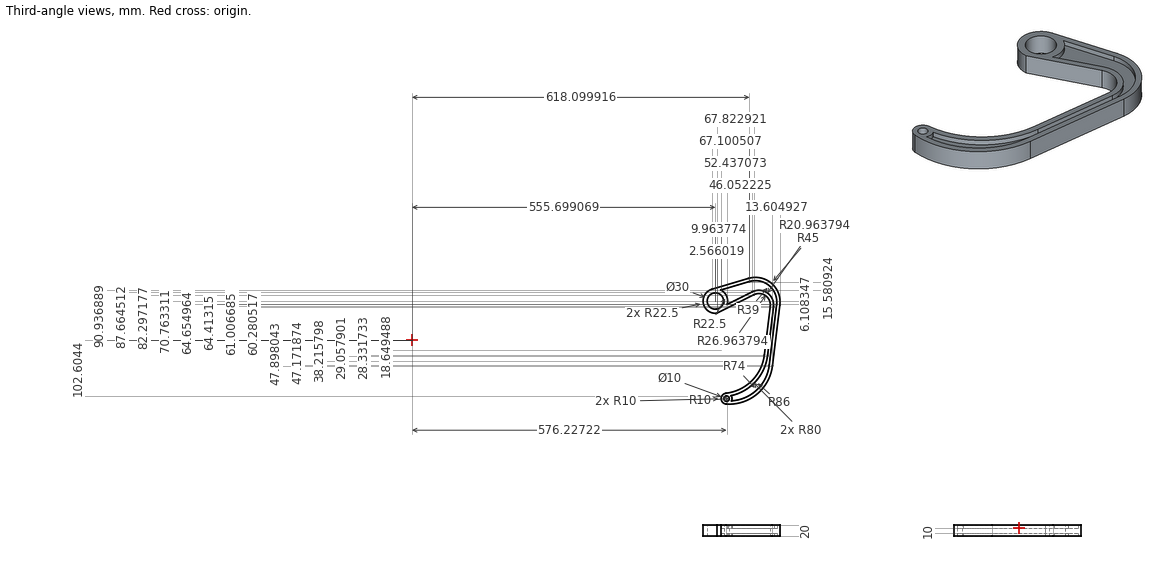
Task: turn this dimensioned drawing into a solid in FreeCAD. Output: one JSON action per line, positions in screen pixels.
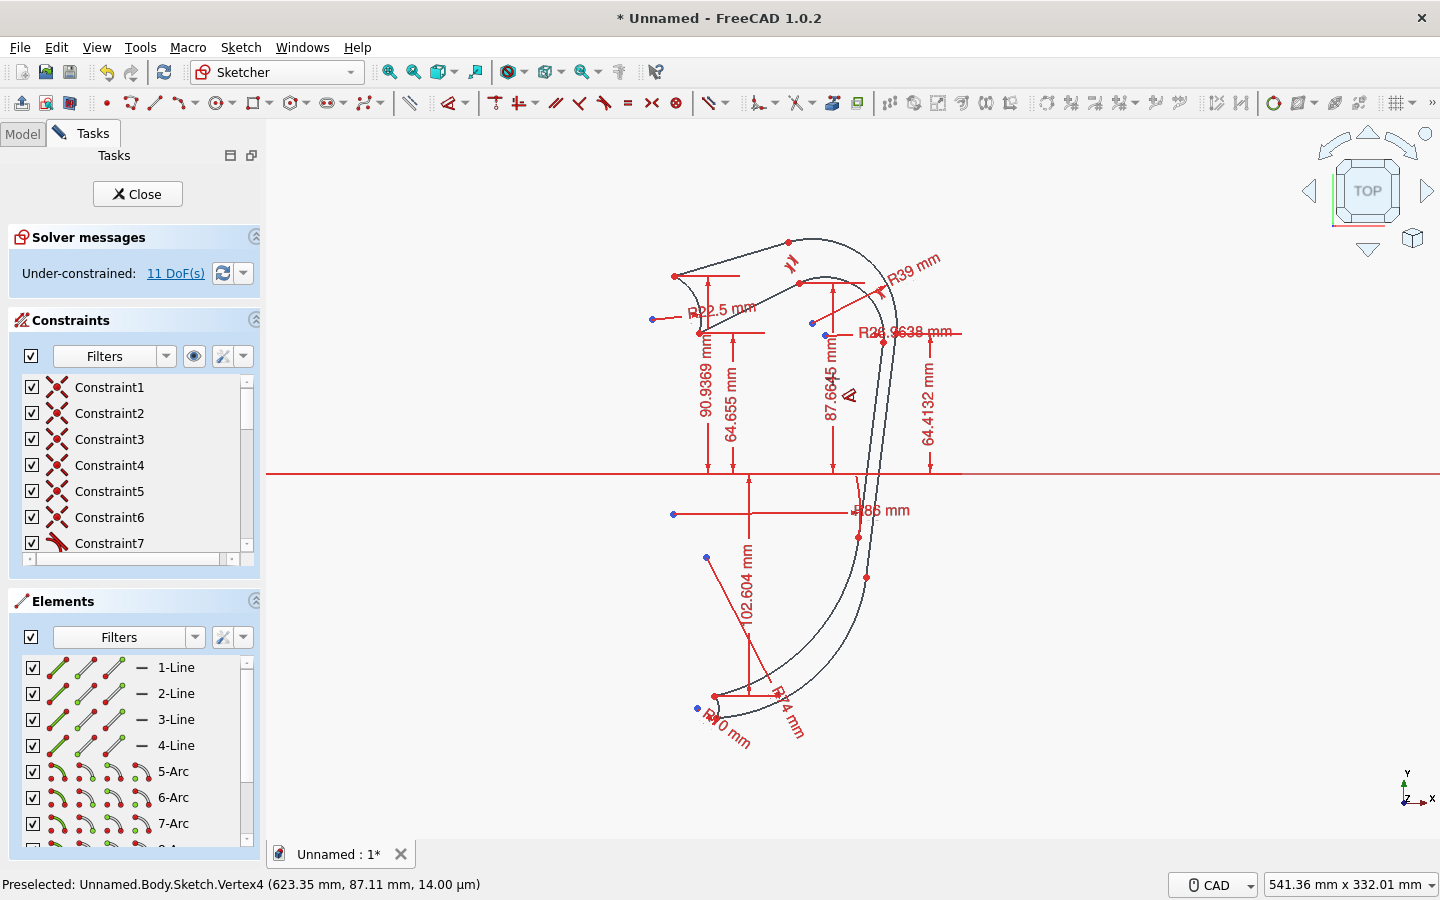
{"action": "left_click", "coordinate": [883, 343]}
{"action": "left_click", "coordinate": [917, 378]}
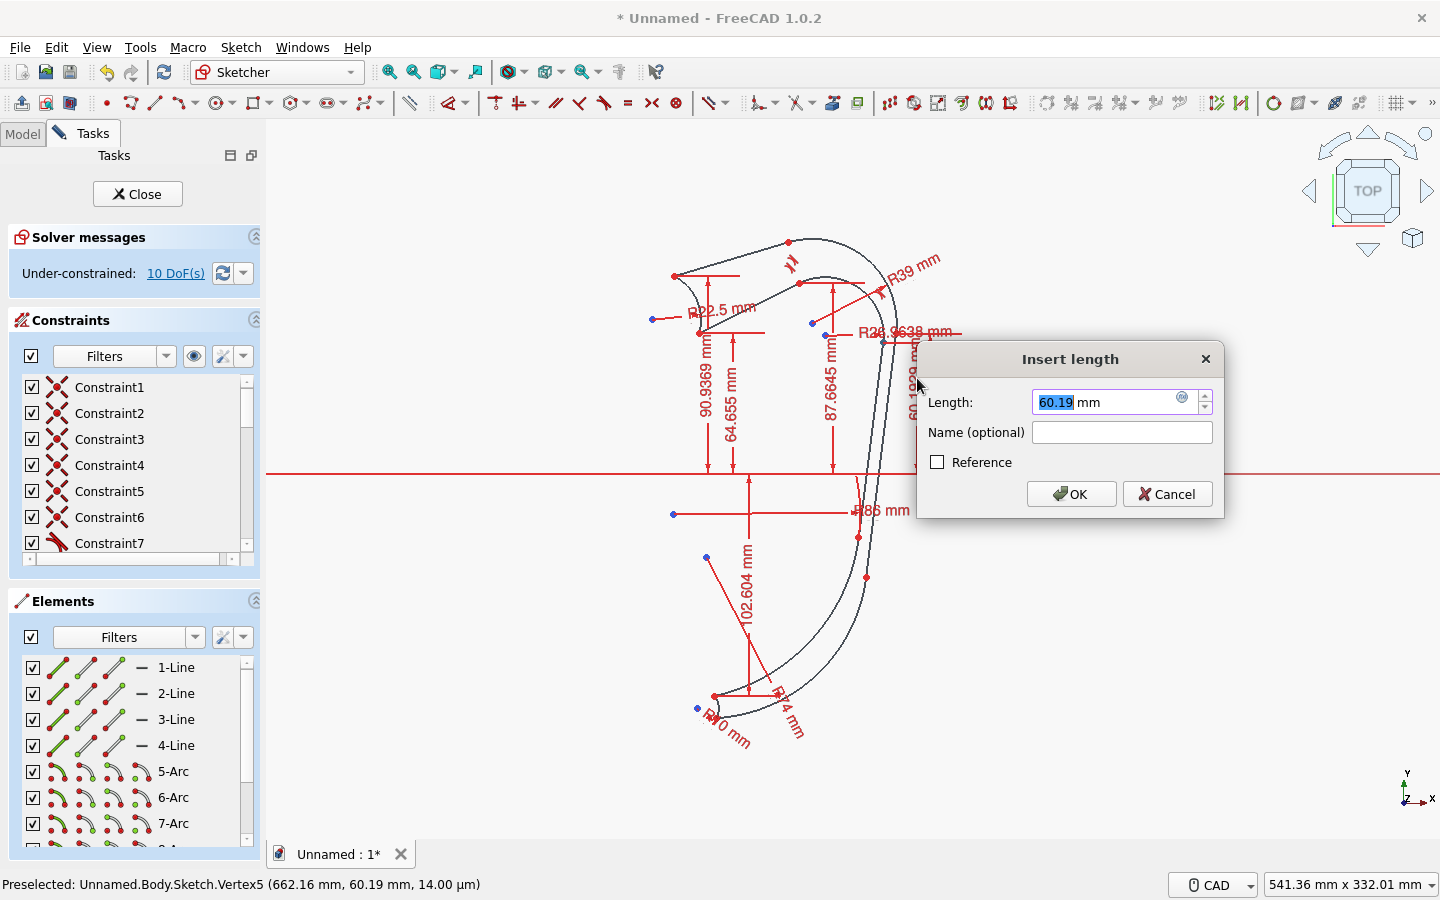
{"action": "type", "text": "60.280517"}
{"action": "key", "text": "Return"}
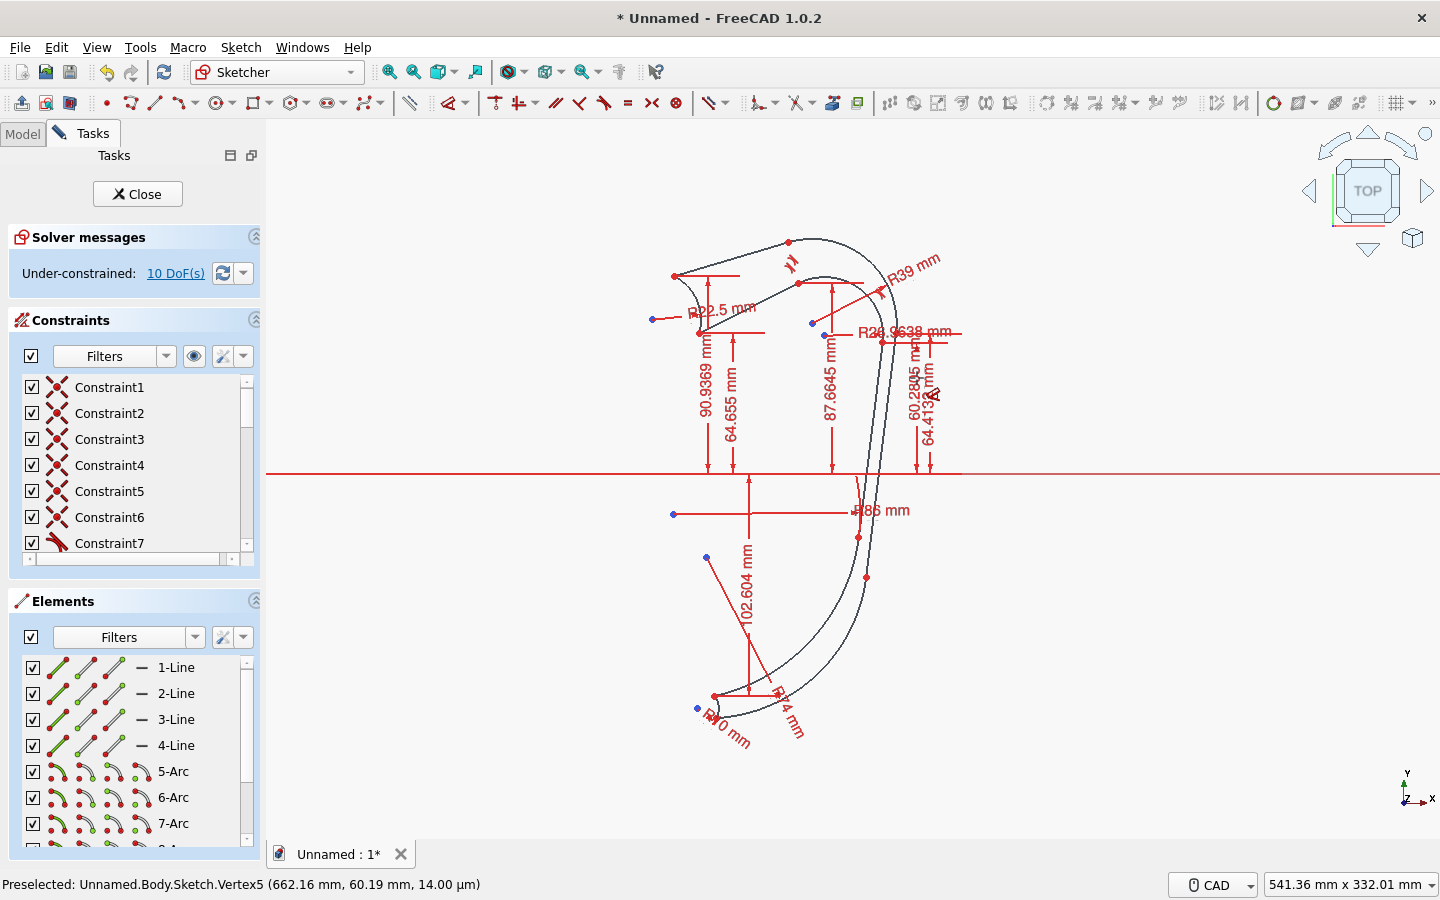
{"action": "left_click", "coordinate": [859, 537]}
{"action": "left_click", "coordinate": [893, 491]}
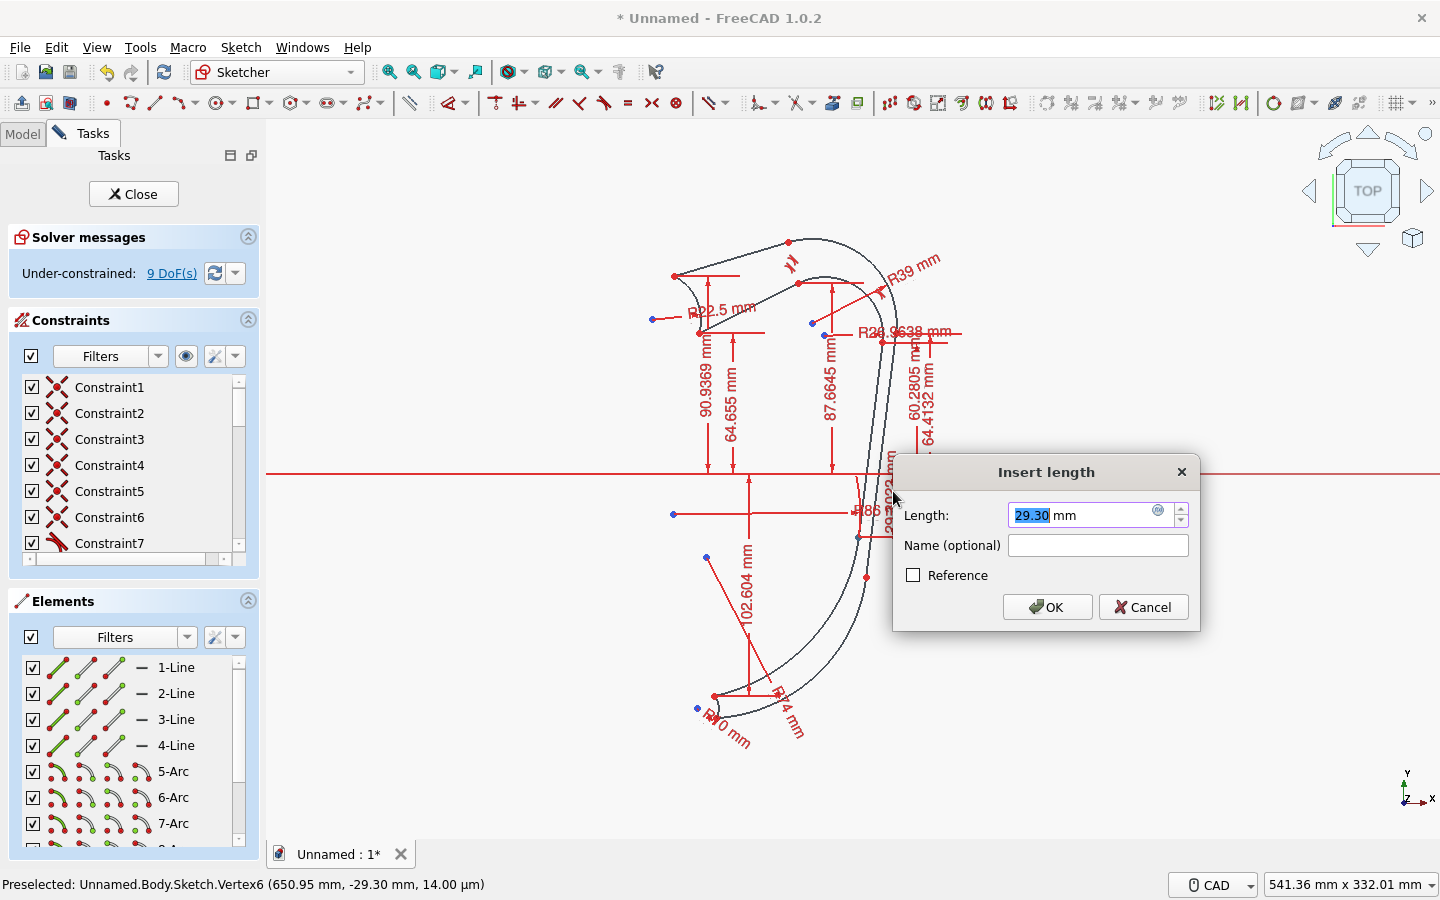
{"action": "type", "text": "29.057901"}
{"action": "key", "text": "Return"}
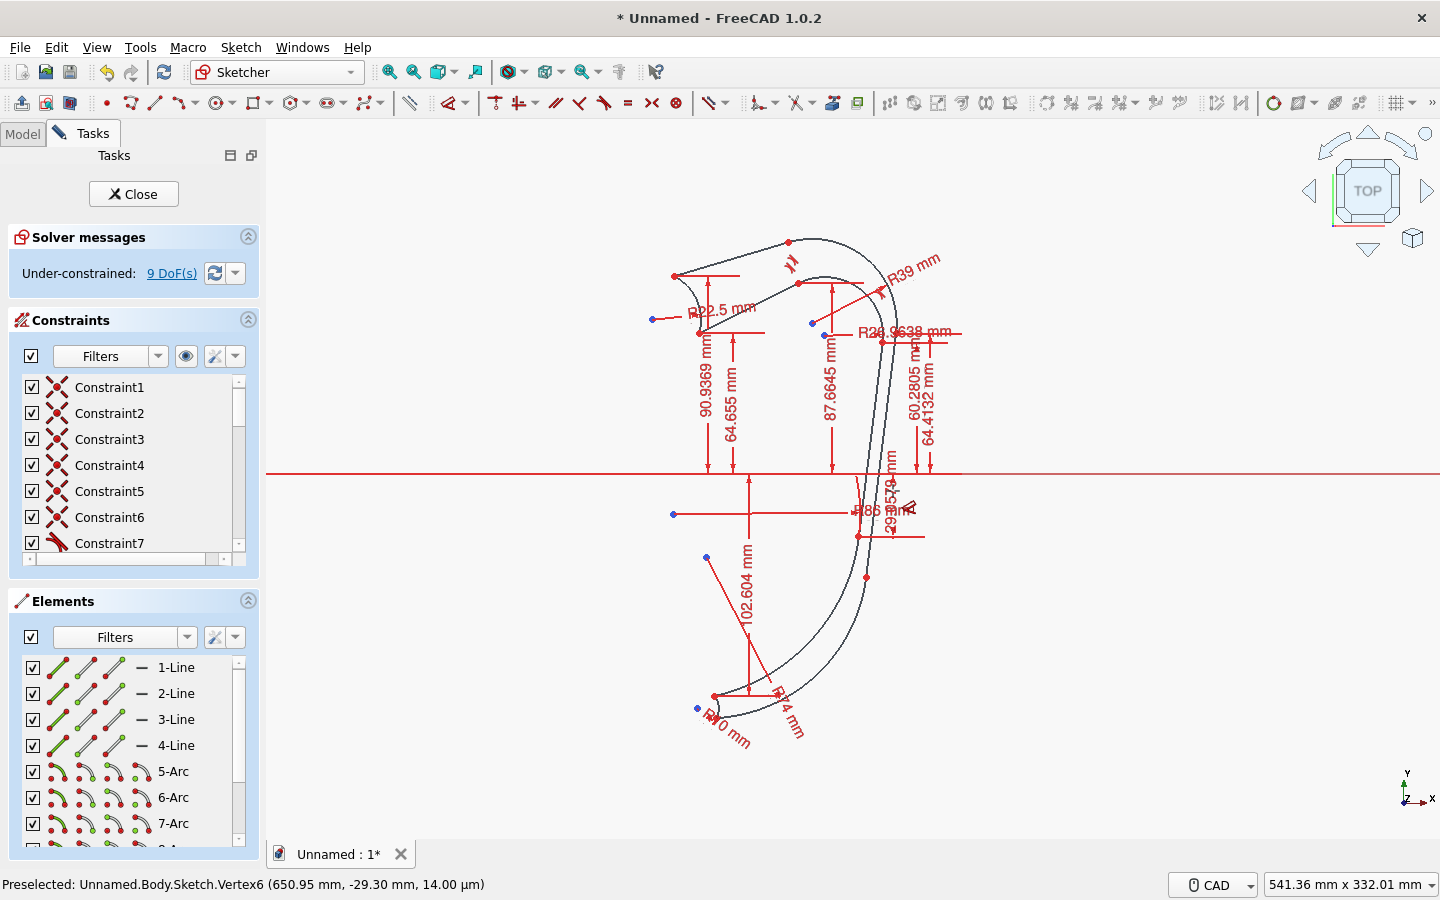
{"action": "left_click", "coordinate": [866, 577]}
{"action": "left_click", "coordinate": [900, 549]}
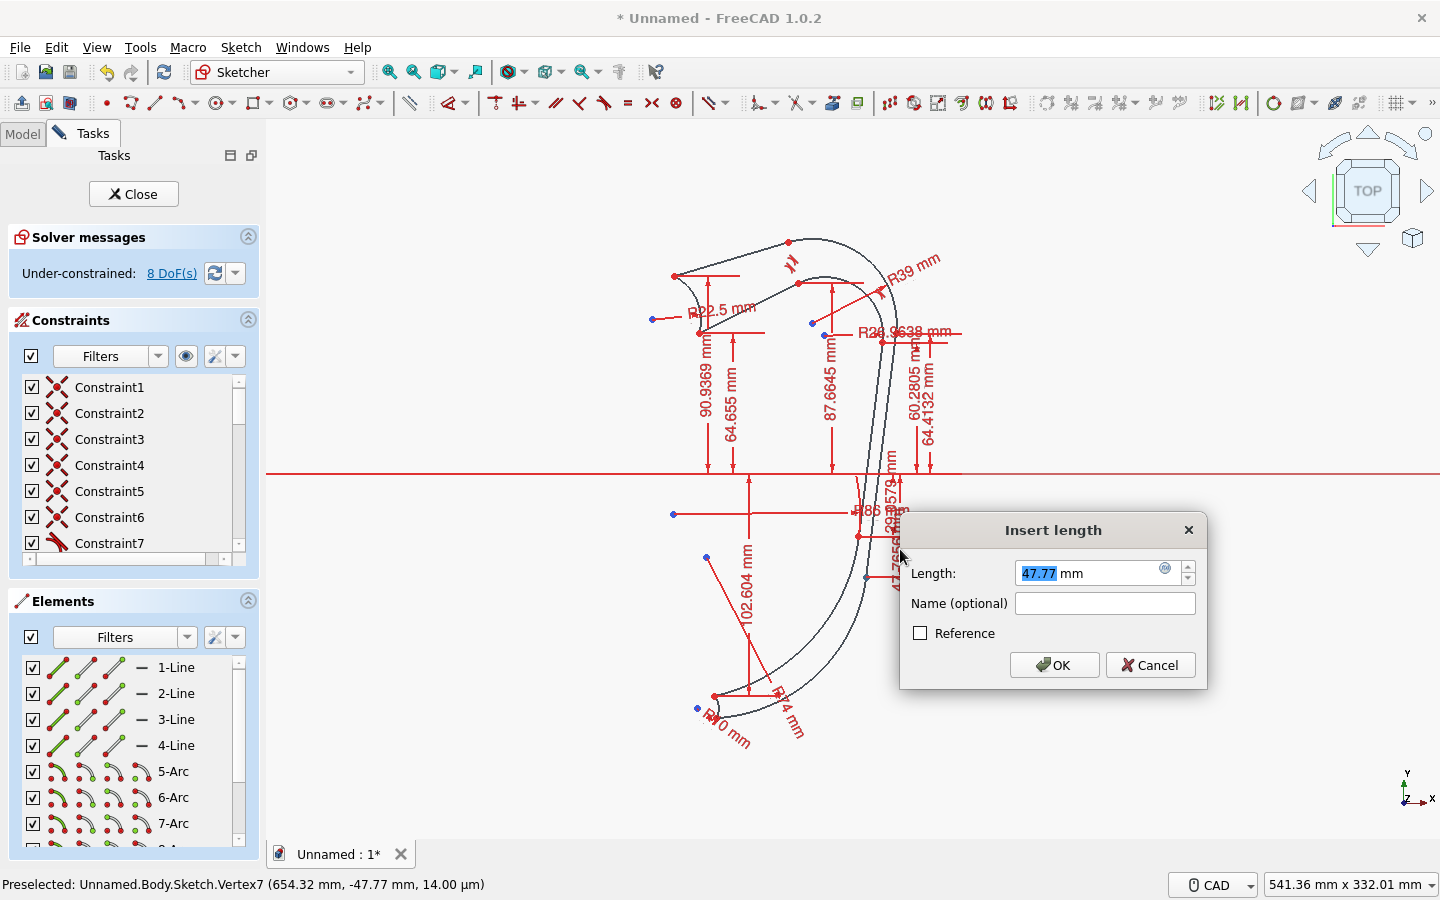
{"action": "type", "text": "47.171874"}
{"action": "key", "text": "Return"}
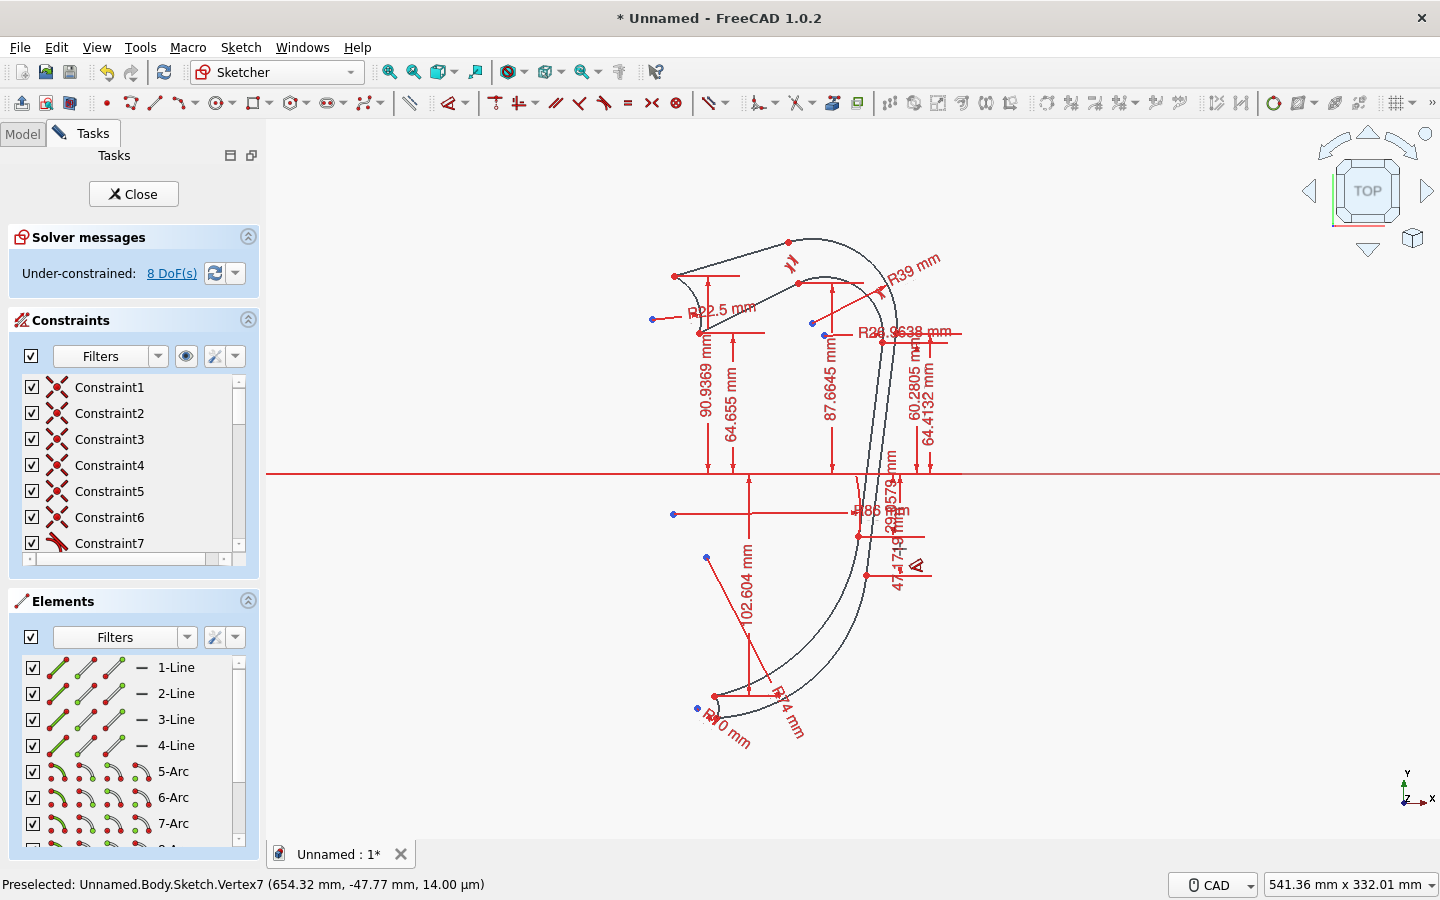
{"action": "left_click", "coordinate": [754, 253]}
{"action": "left_click", "coordinate": [731, 208]}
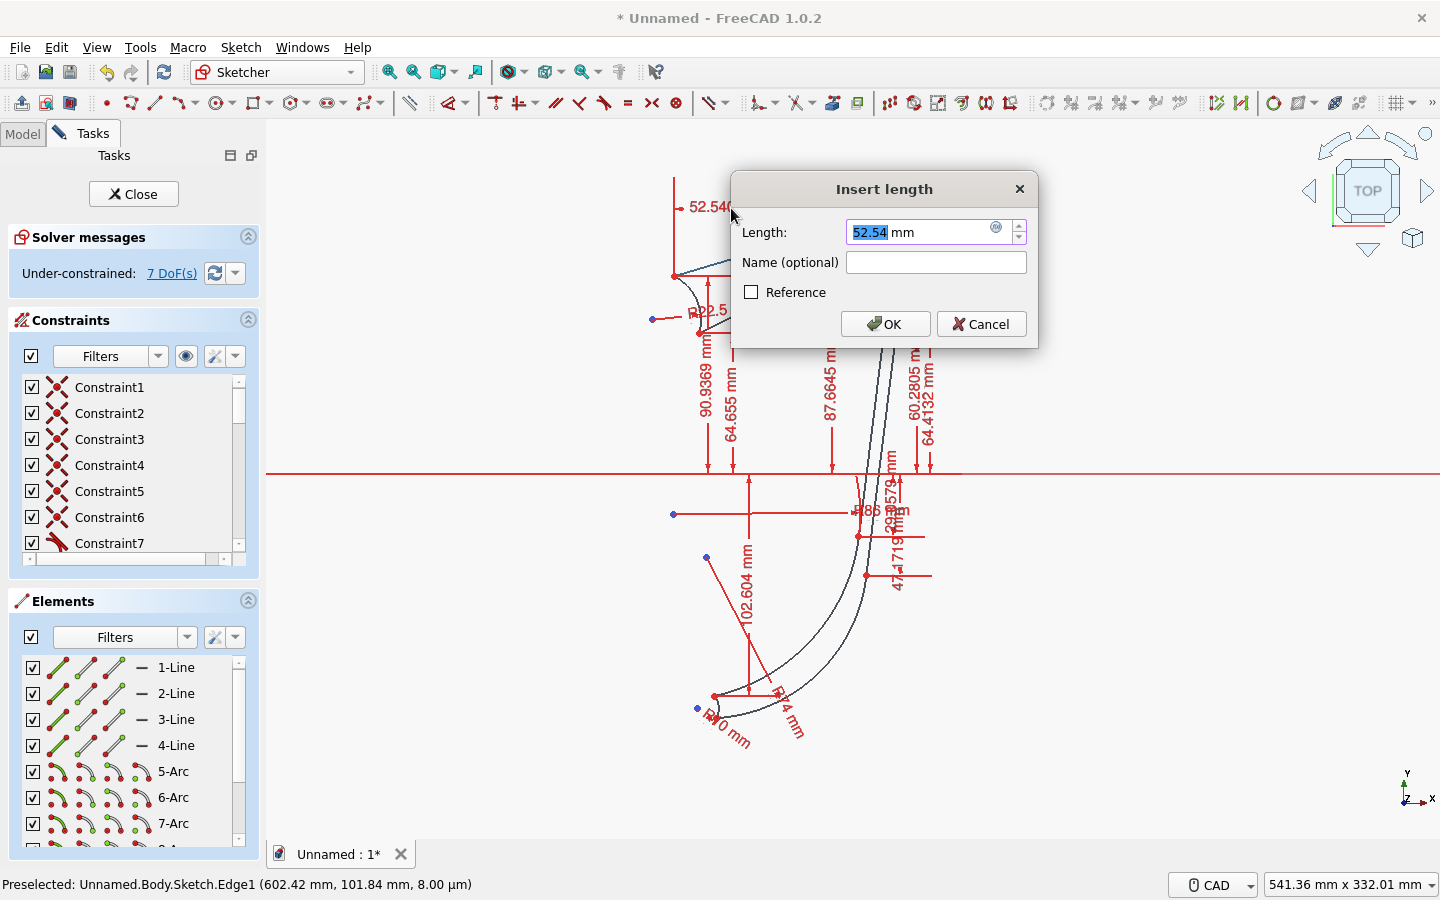
{"action": "type", "text": "52.437073"}
{"action": "key", "text": "Return"}